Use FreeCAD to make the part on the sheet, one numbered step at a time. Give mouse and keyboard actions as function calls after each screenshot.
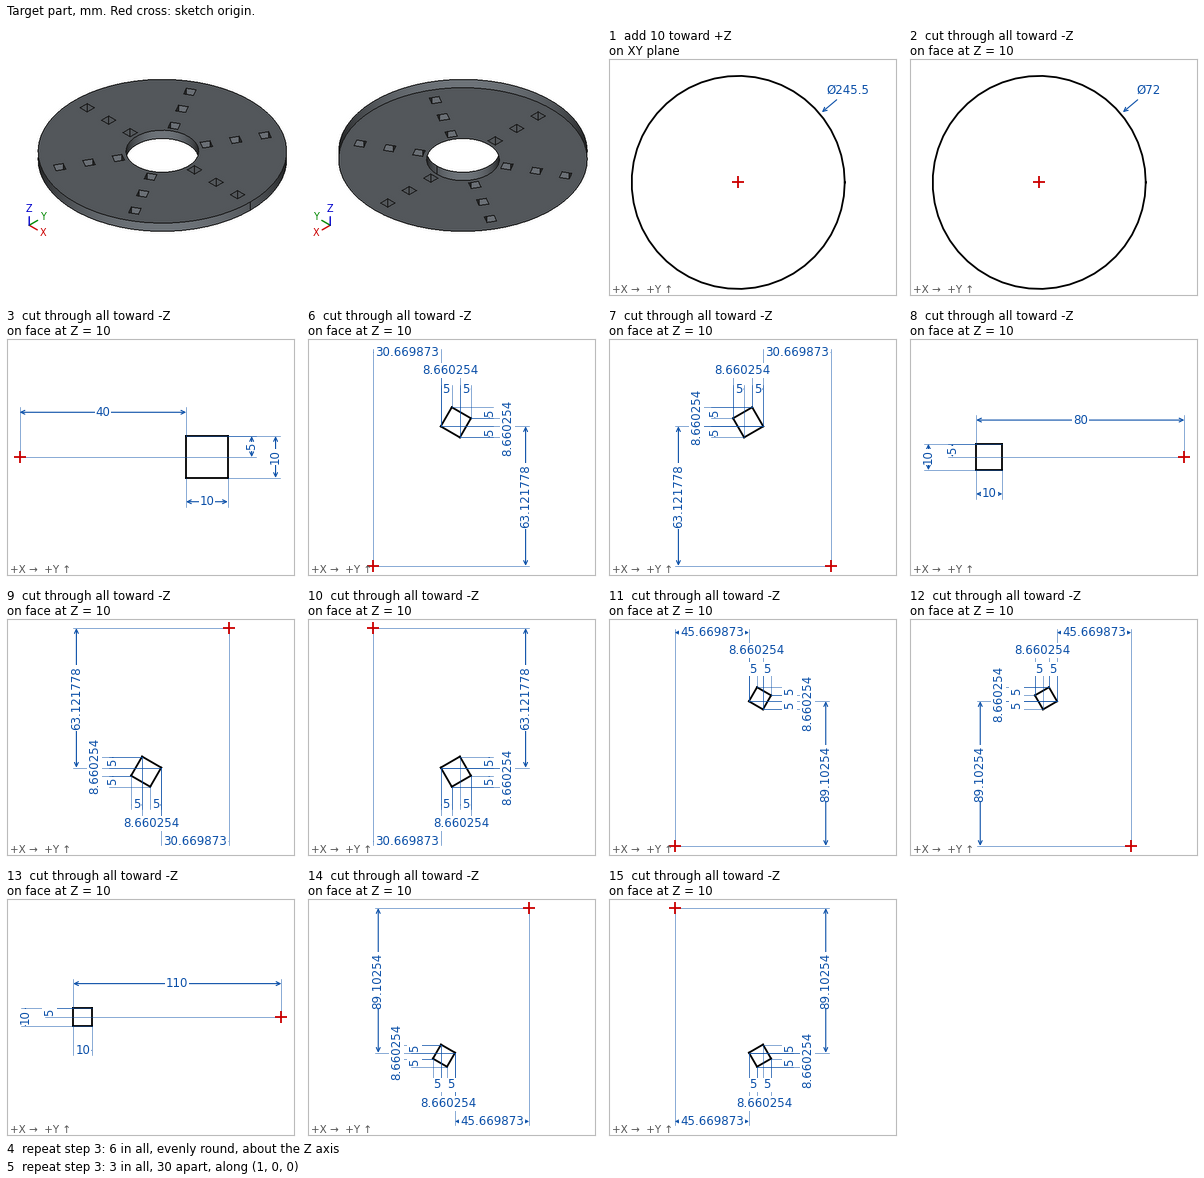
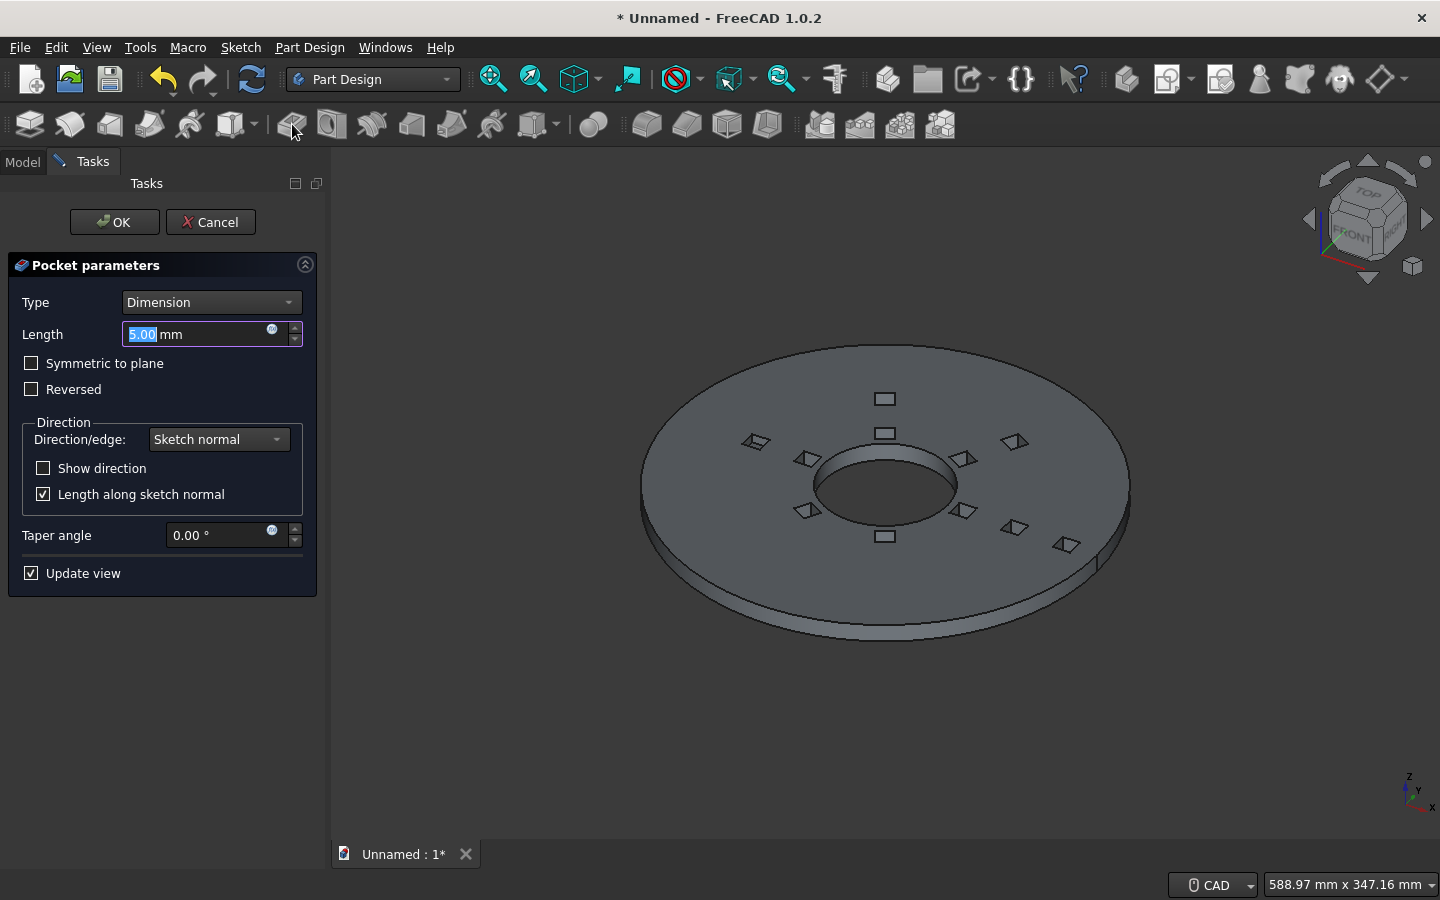
click(212, 302)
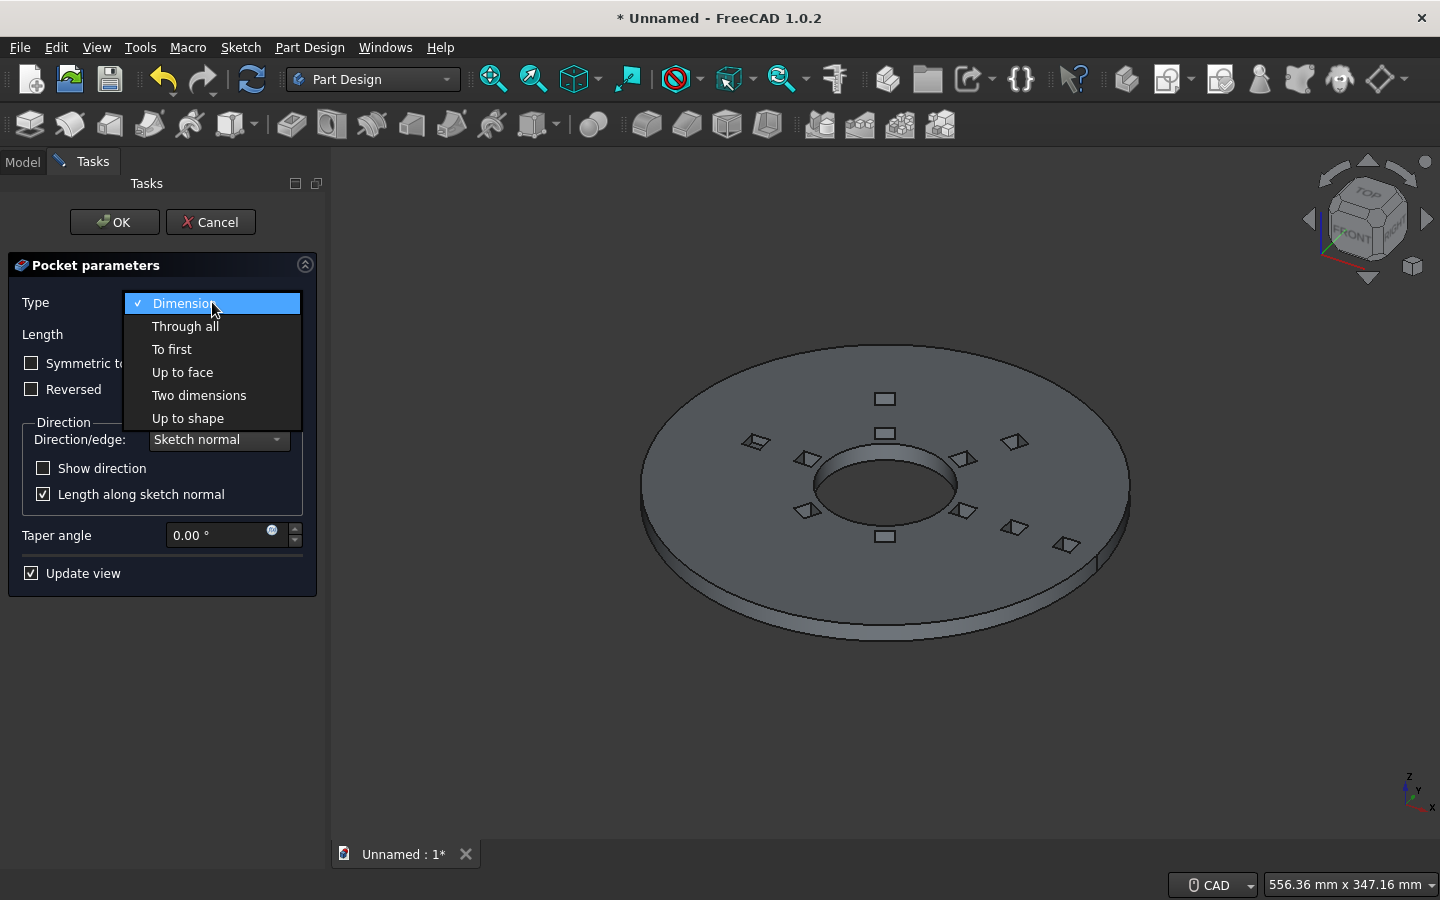
click(212, 326)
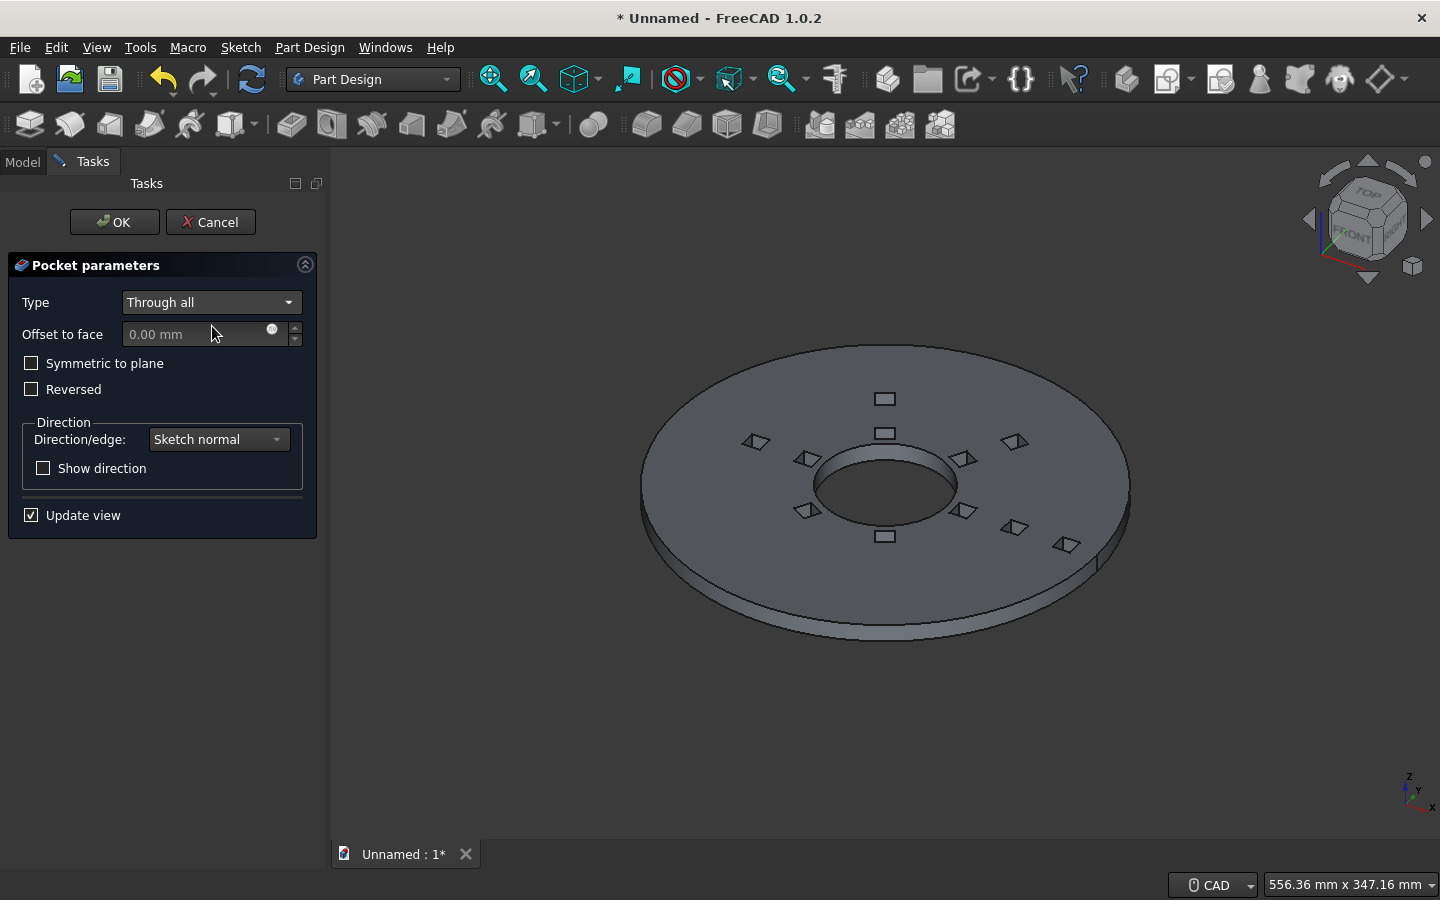
click(115, 222)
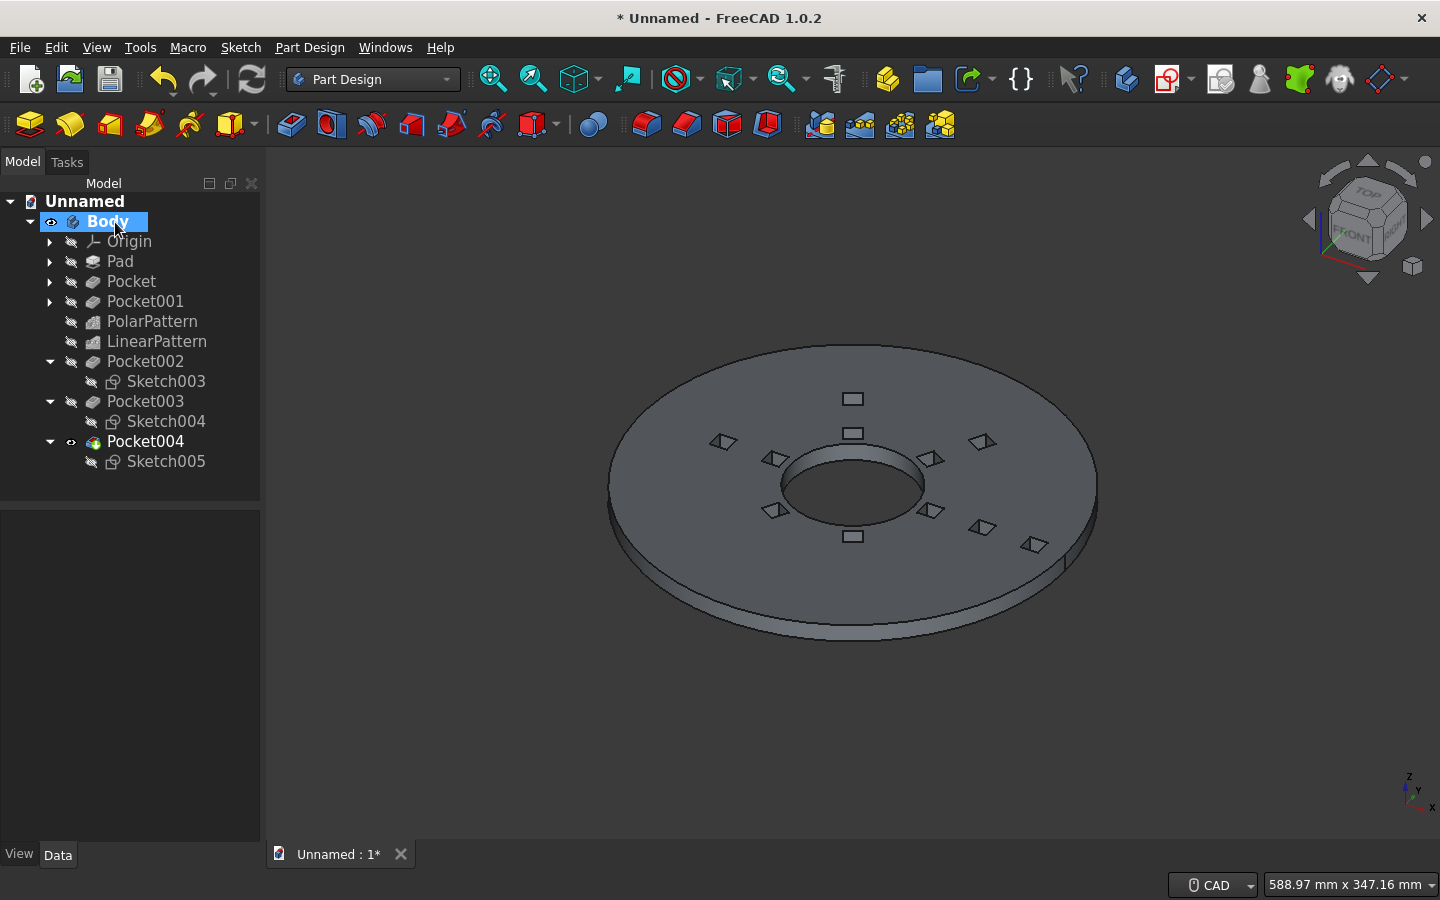
click(783, 553)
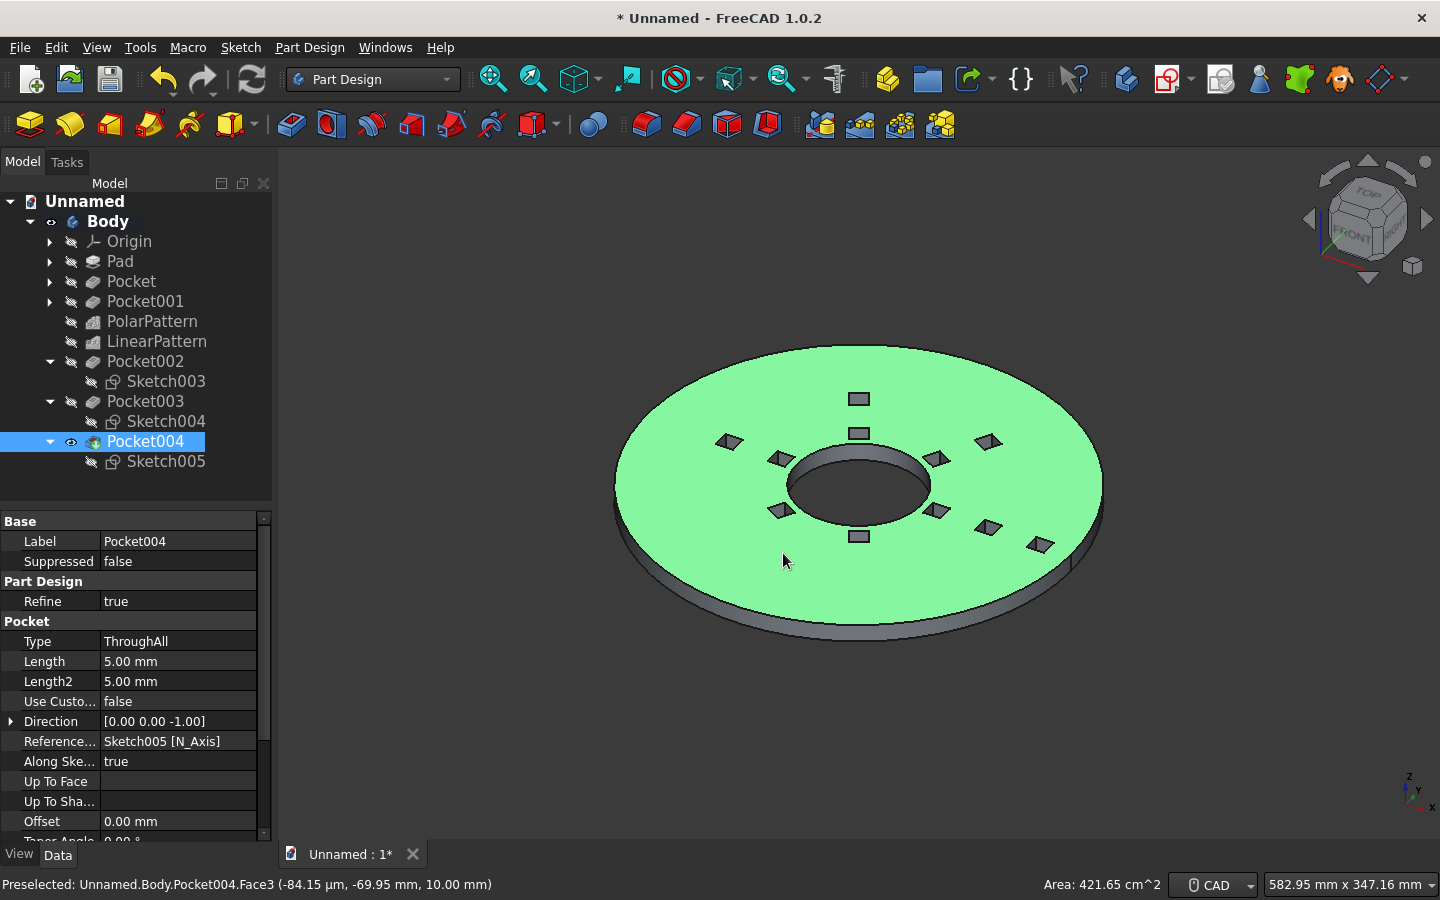
click(1168, 80)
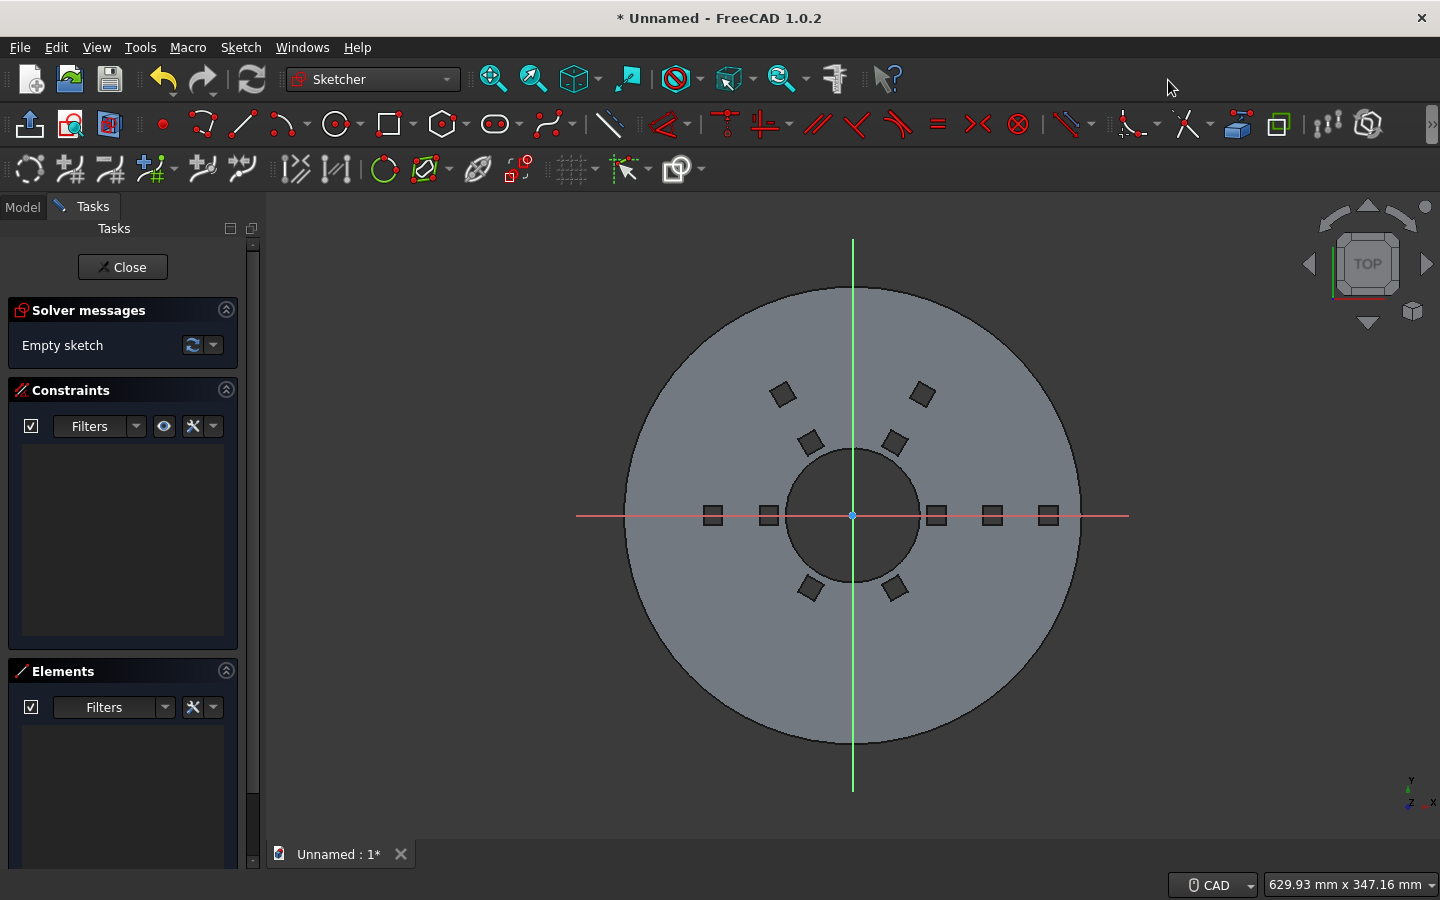
scroll(783, 644, up, 14)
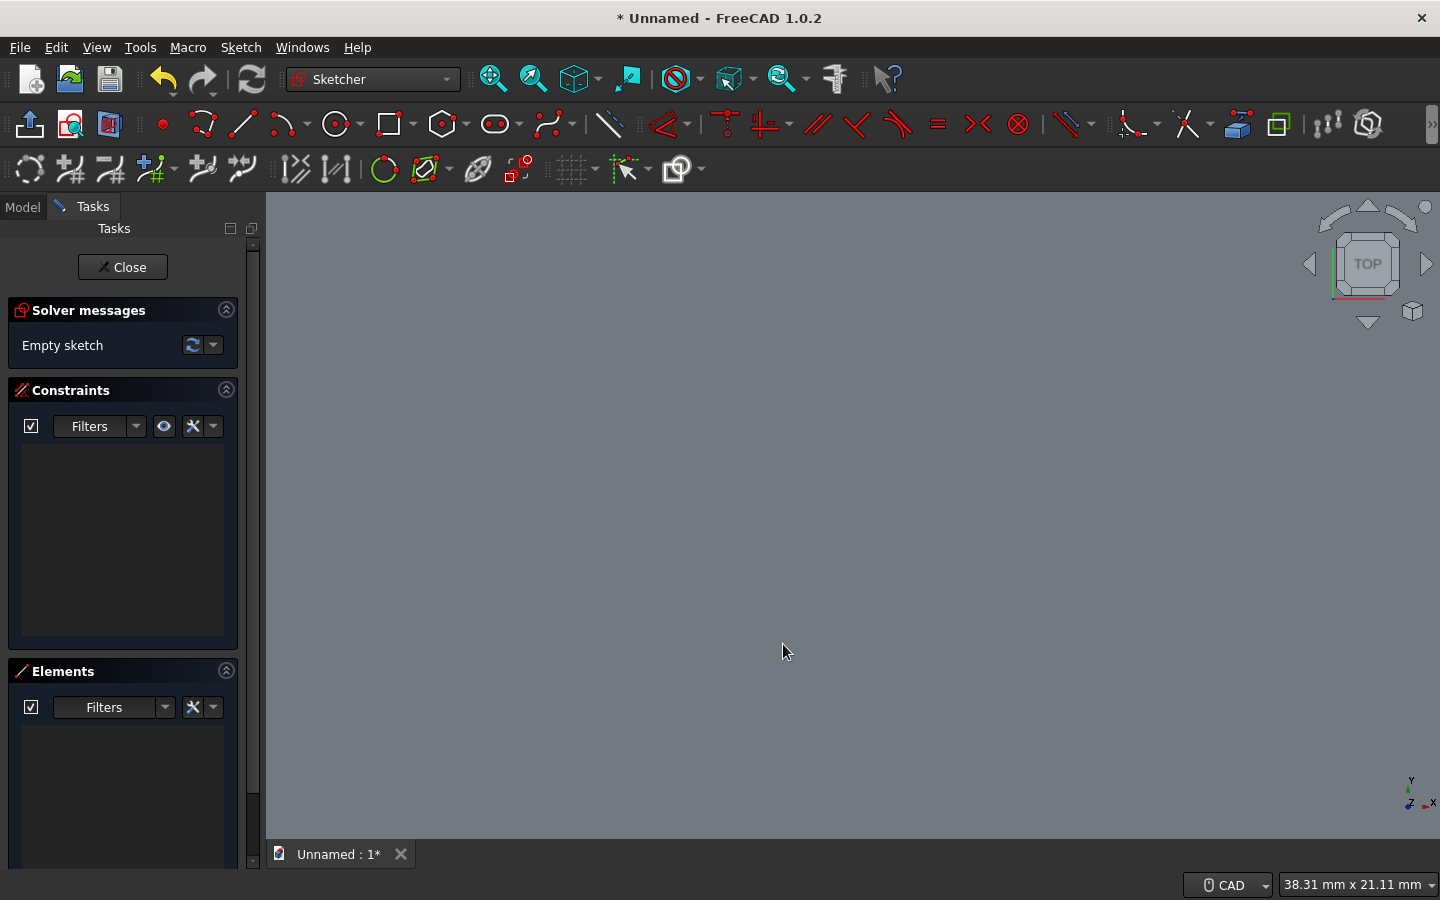
key(g)
key(m)